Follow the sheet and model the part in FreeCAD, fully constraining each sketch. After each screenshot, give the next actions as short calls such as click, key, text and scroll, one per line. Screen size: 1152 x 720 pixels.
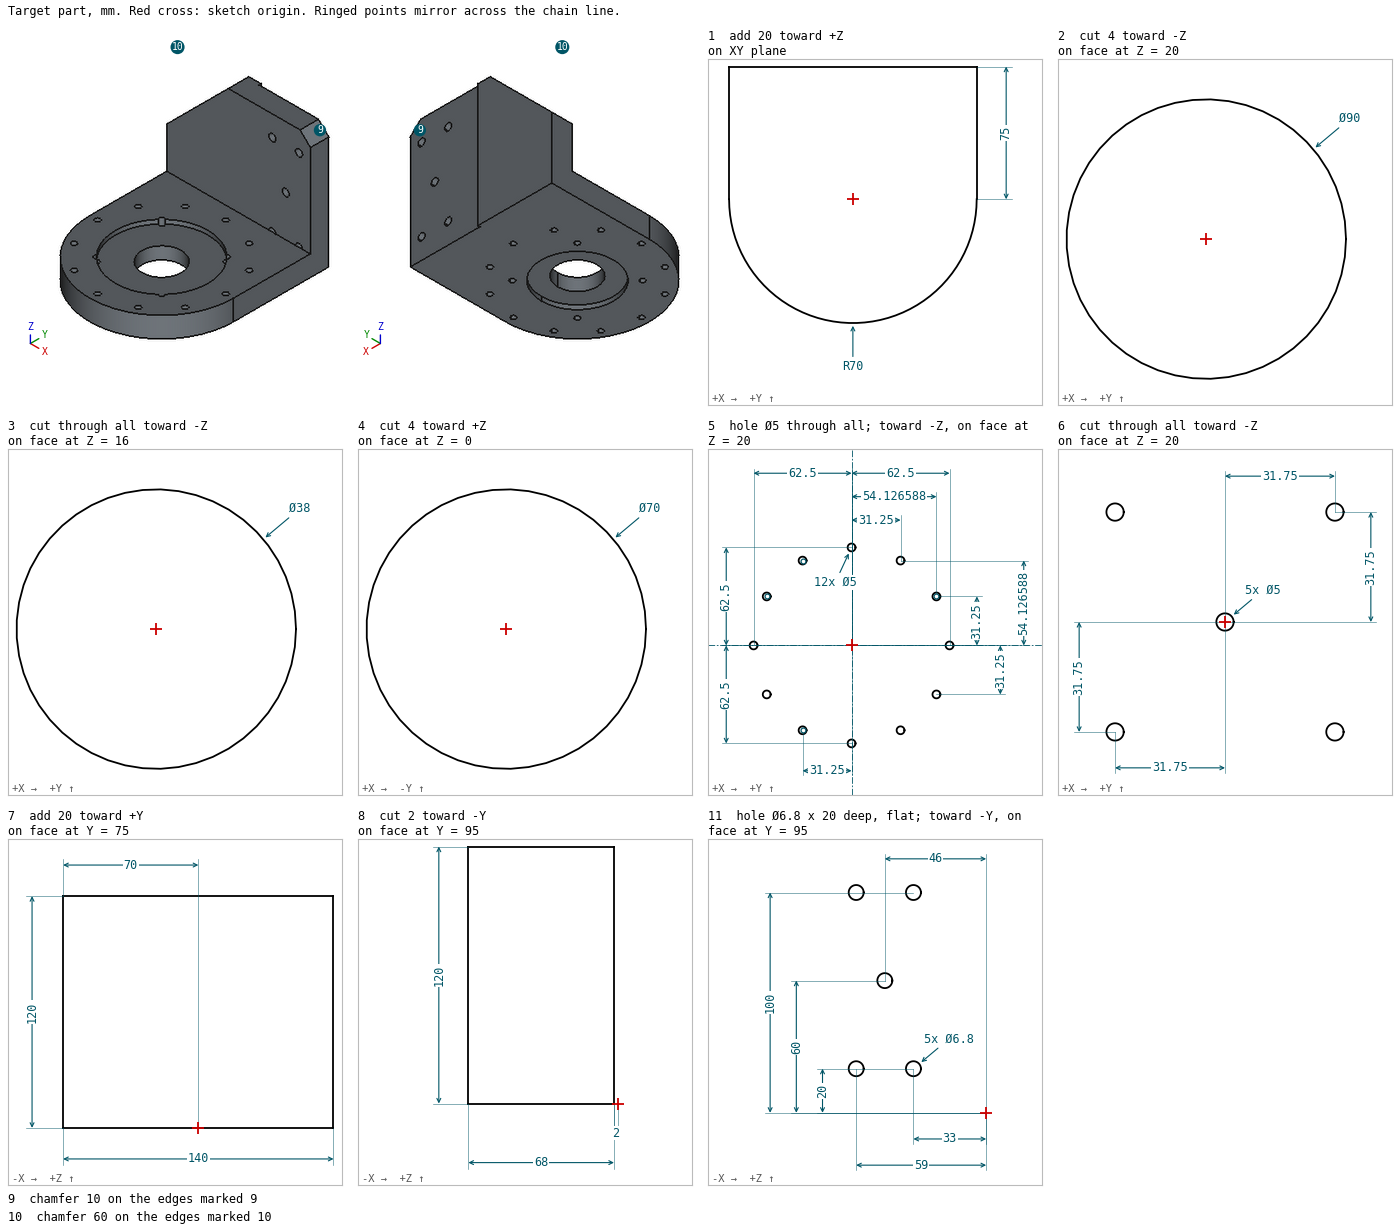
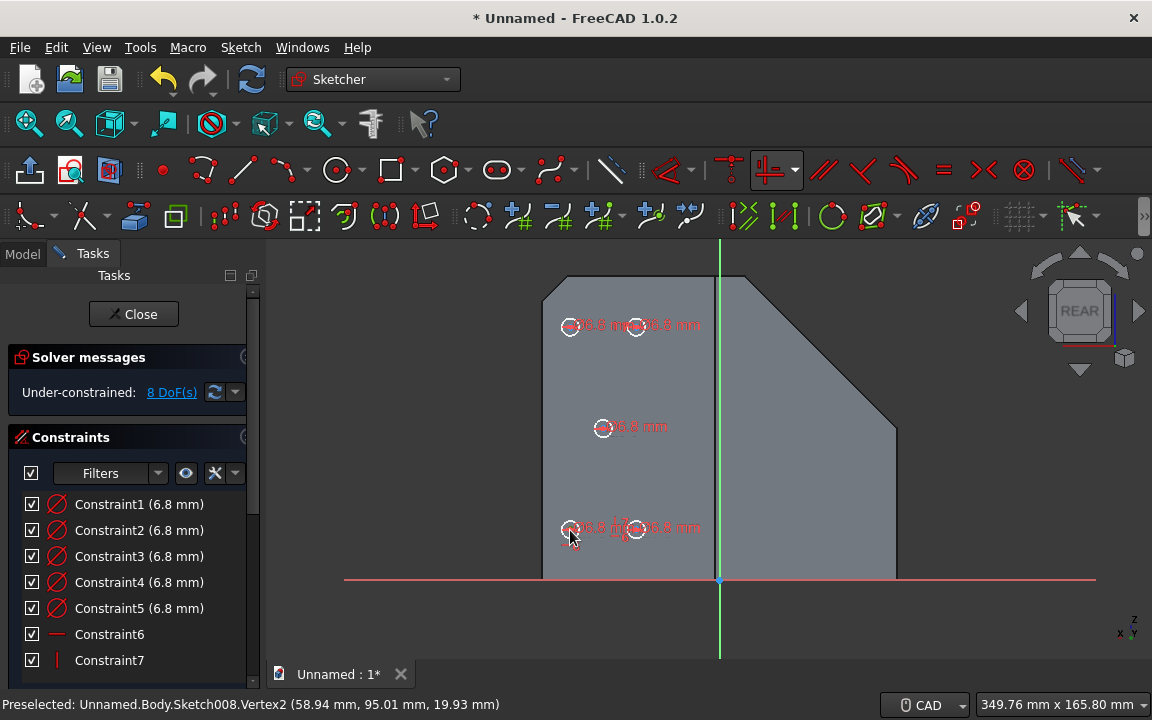
click(570, 327)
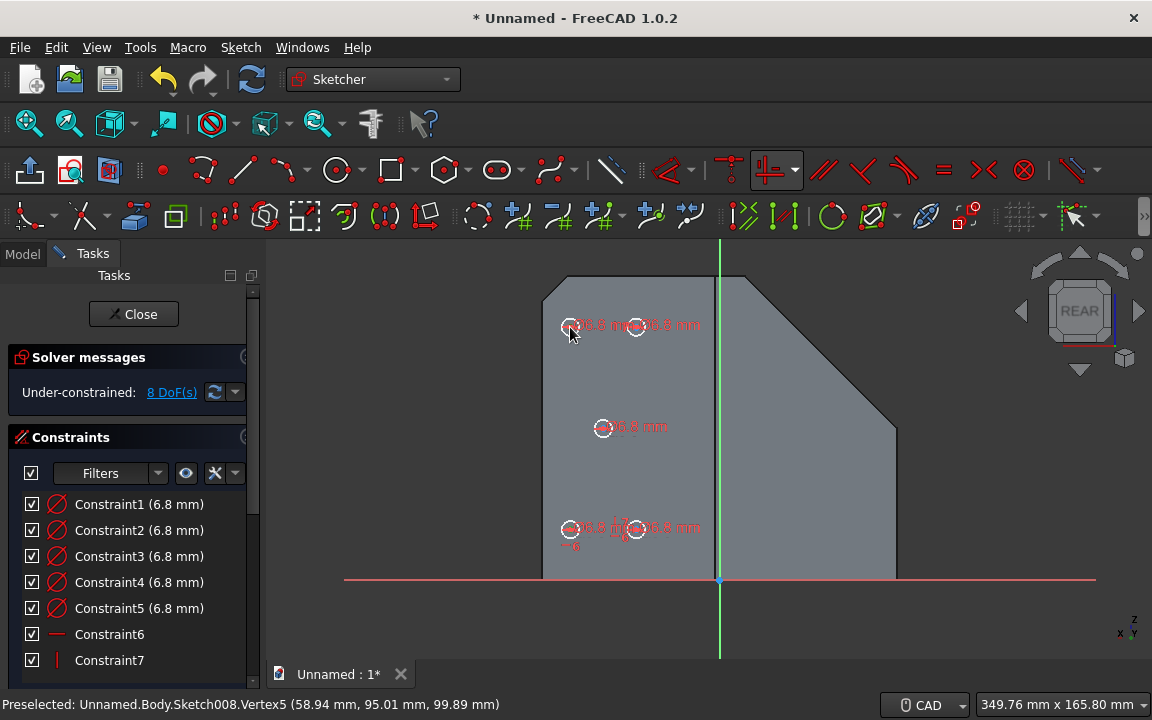
click(798, 170)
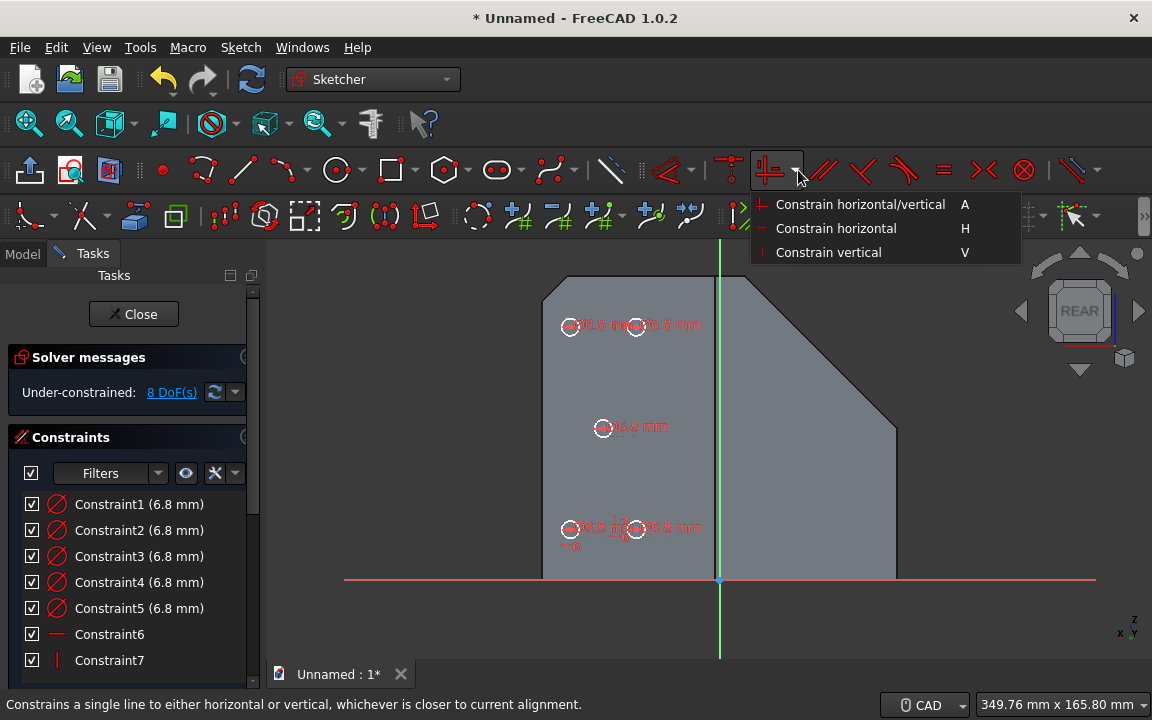
click(886, 252)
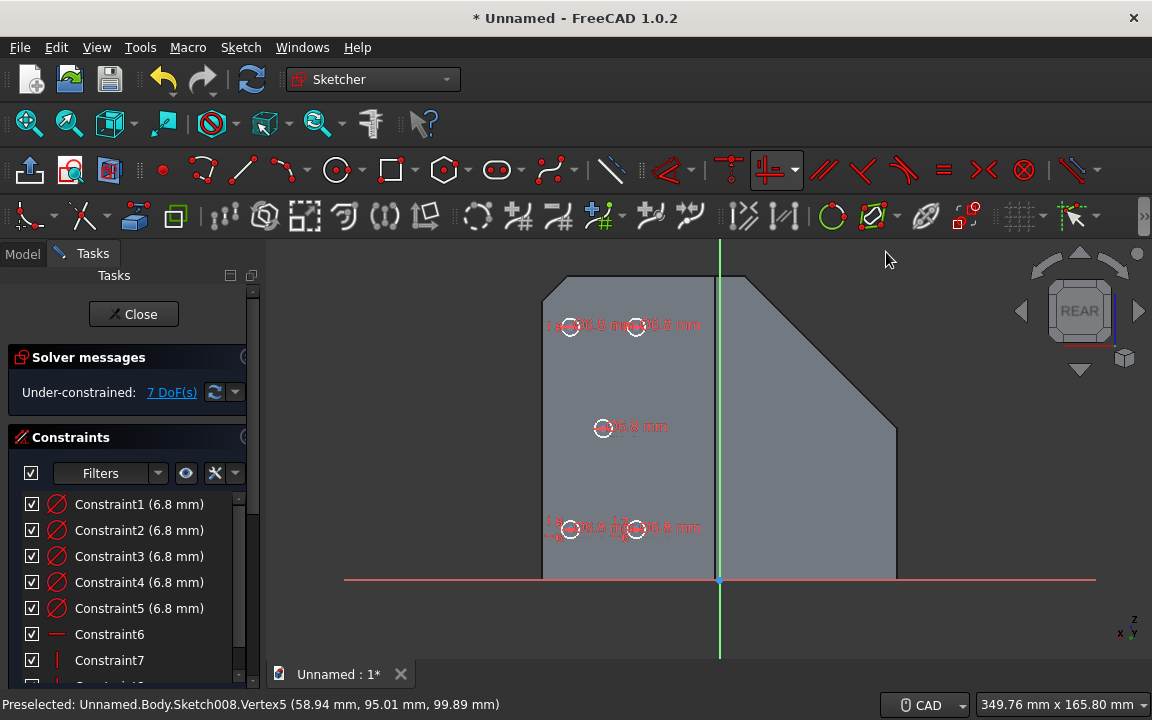
click(636, 327)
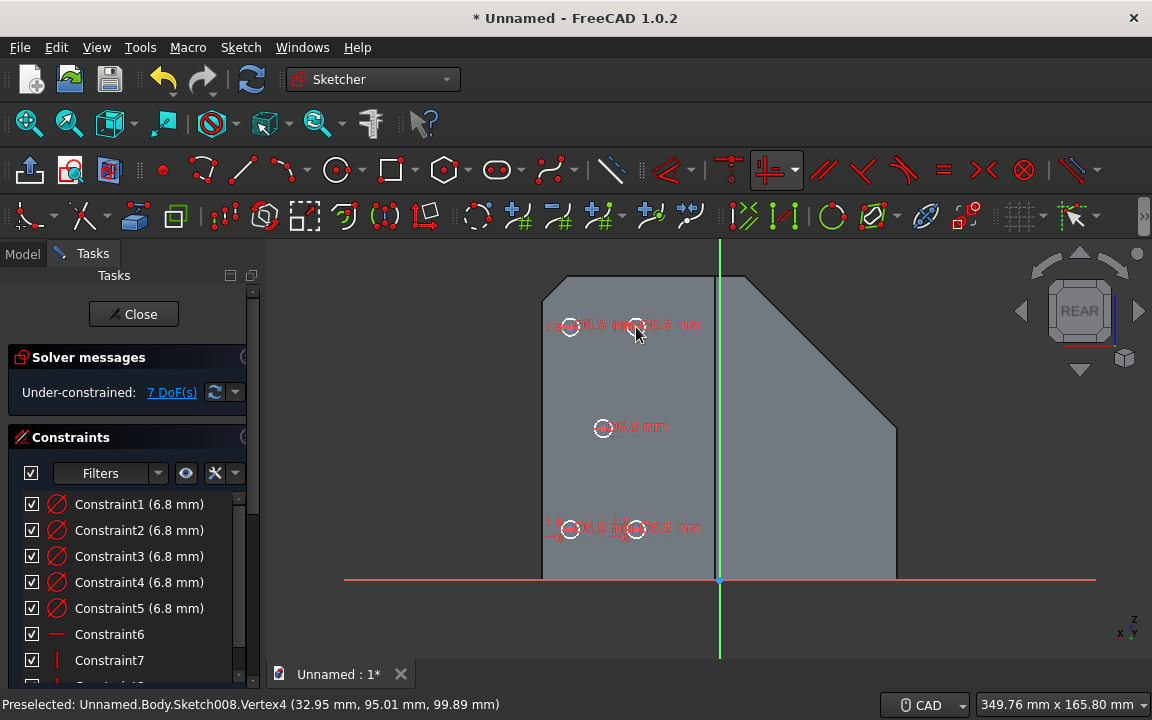
click(570, 327)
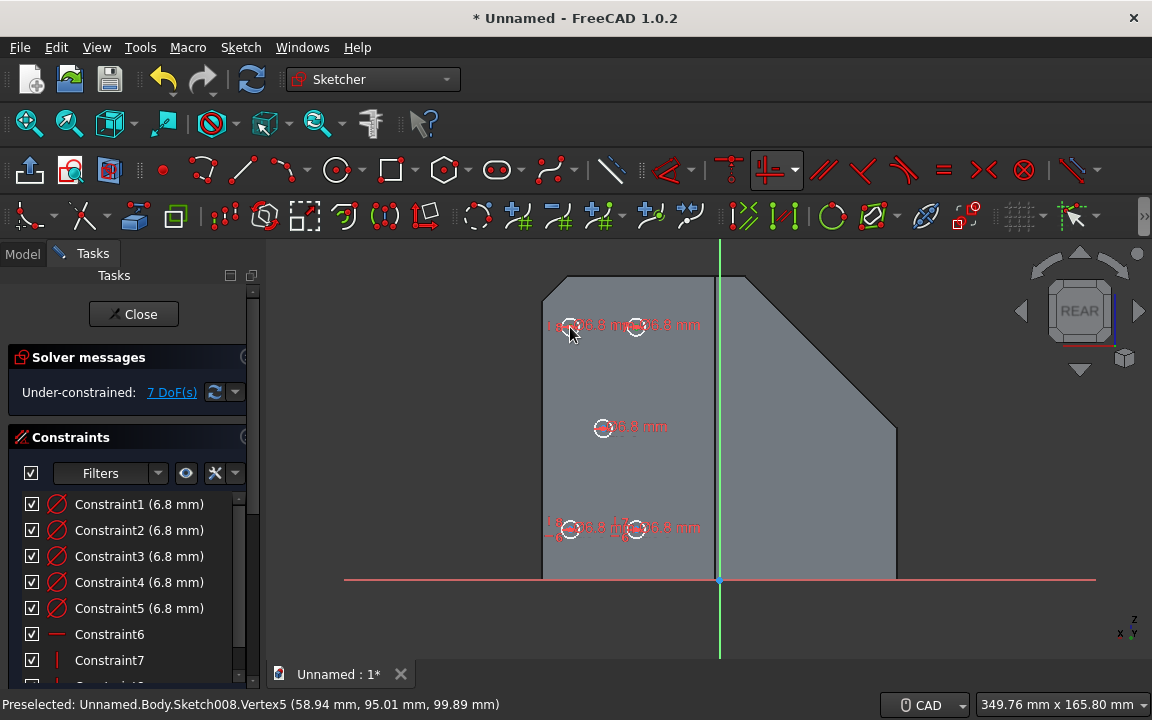
key(h)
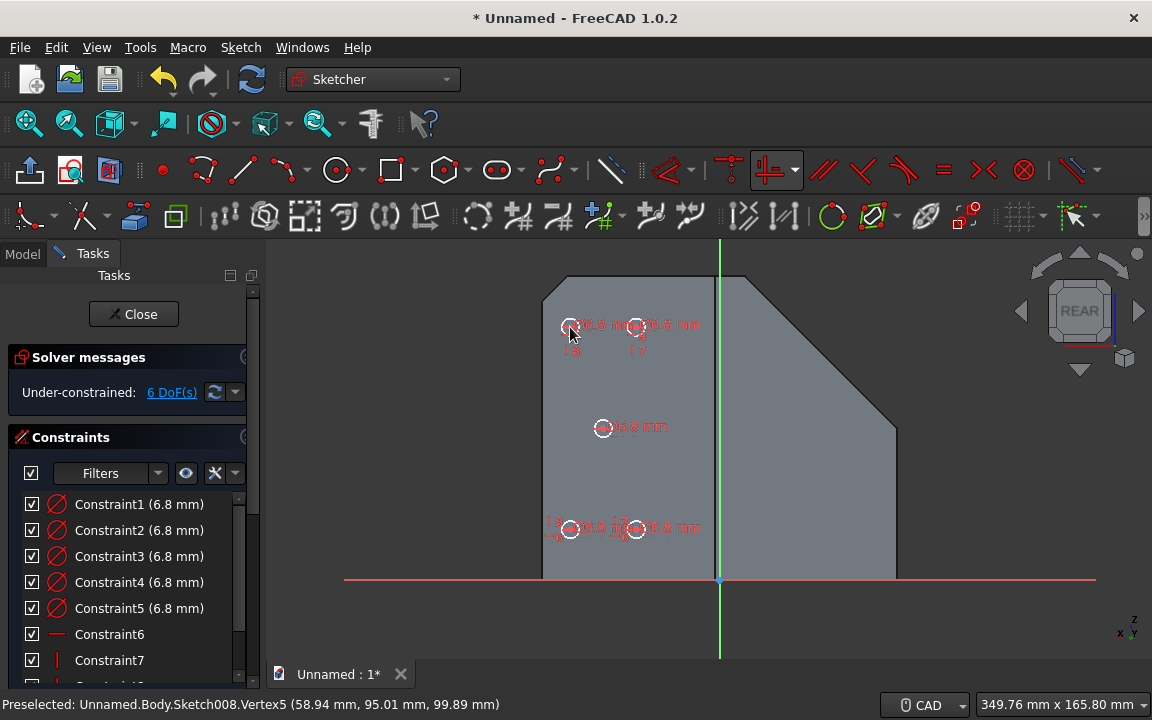
click(666, 170)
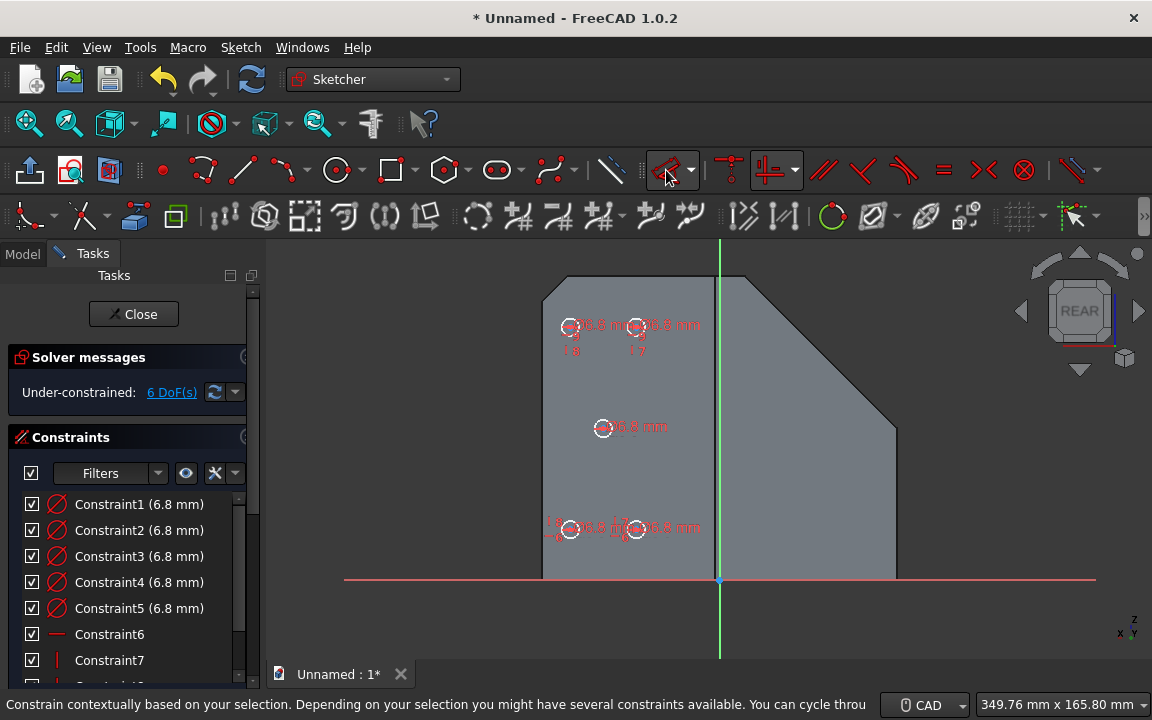
click(636, 530)
click(678, 614)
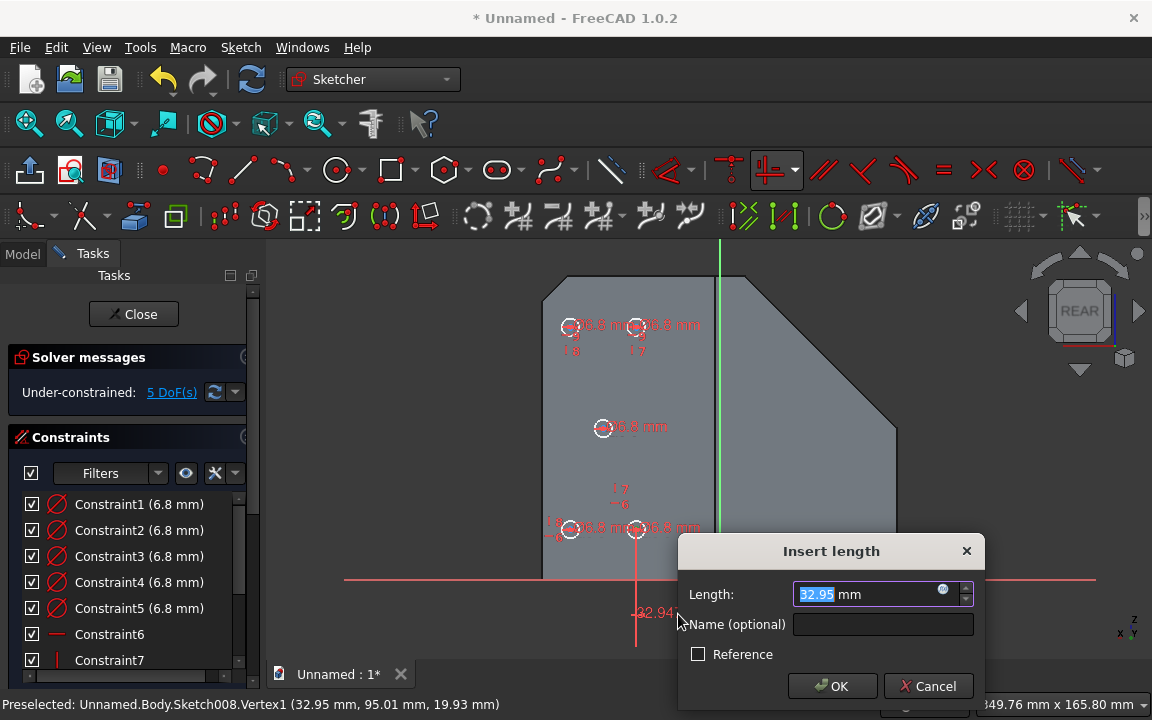
text(33)
key(Return)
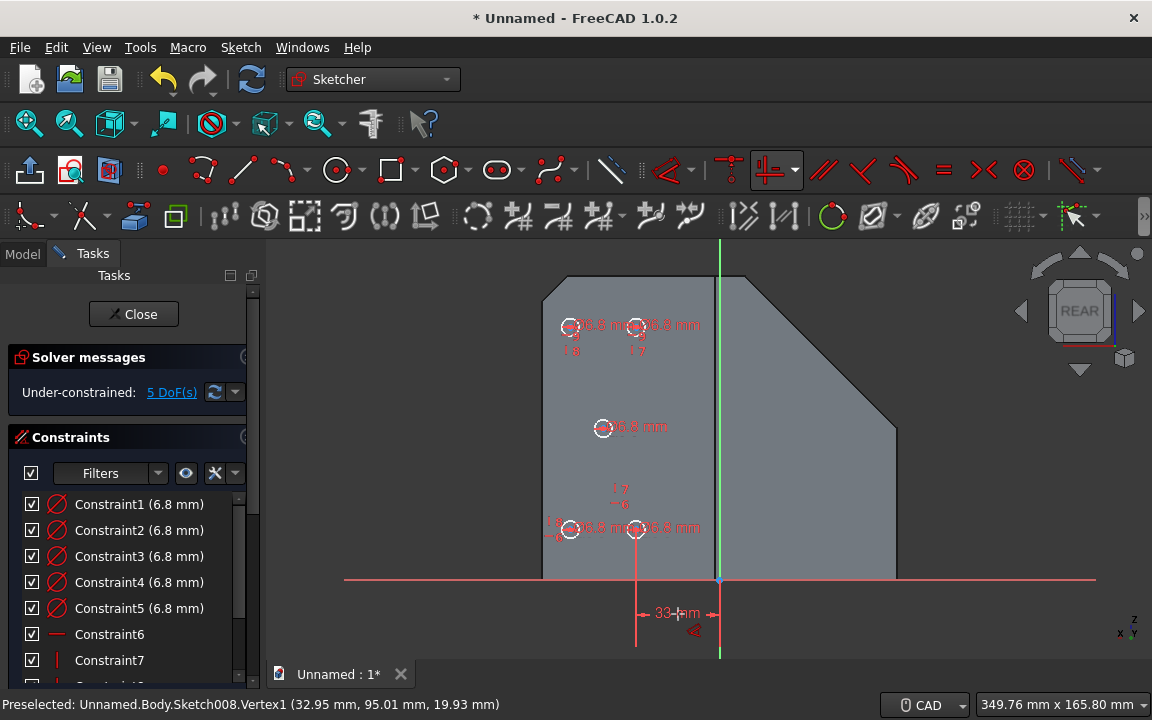
click(636, 530)
click(754, 555)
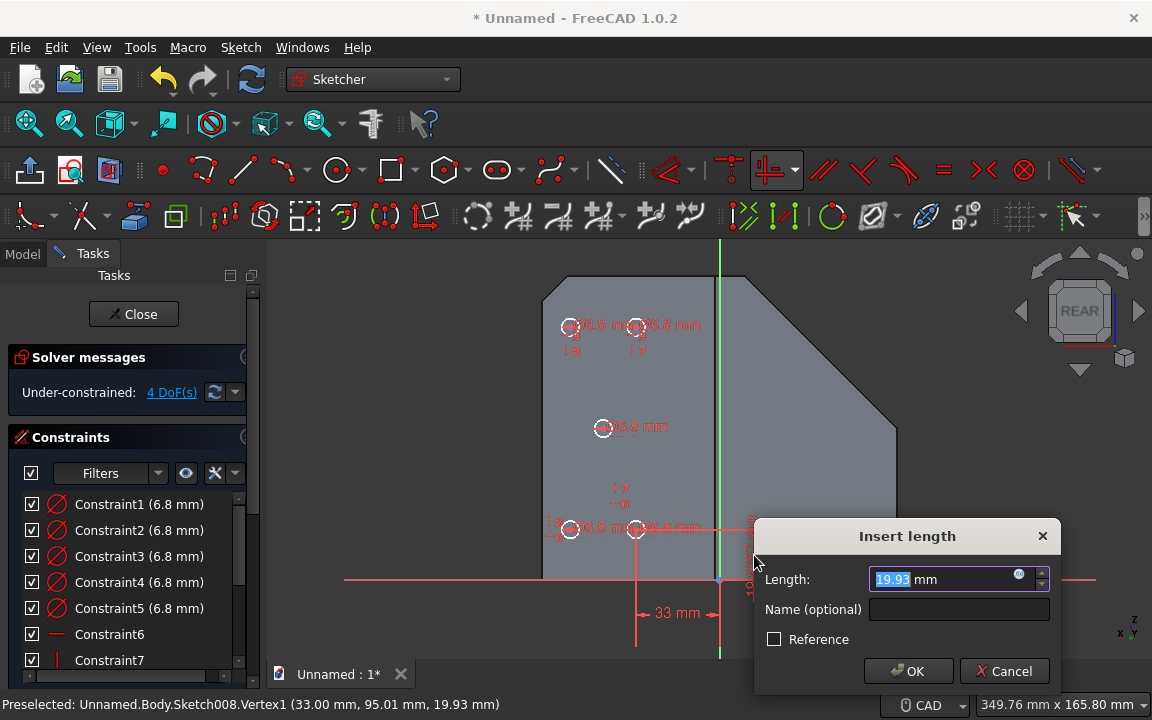
text(20)
key(Return)